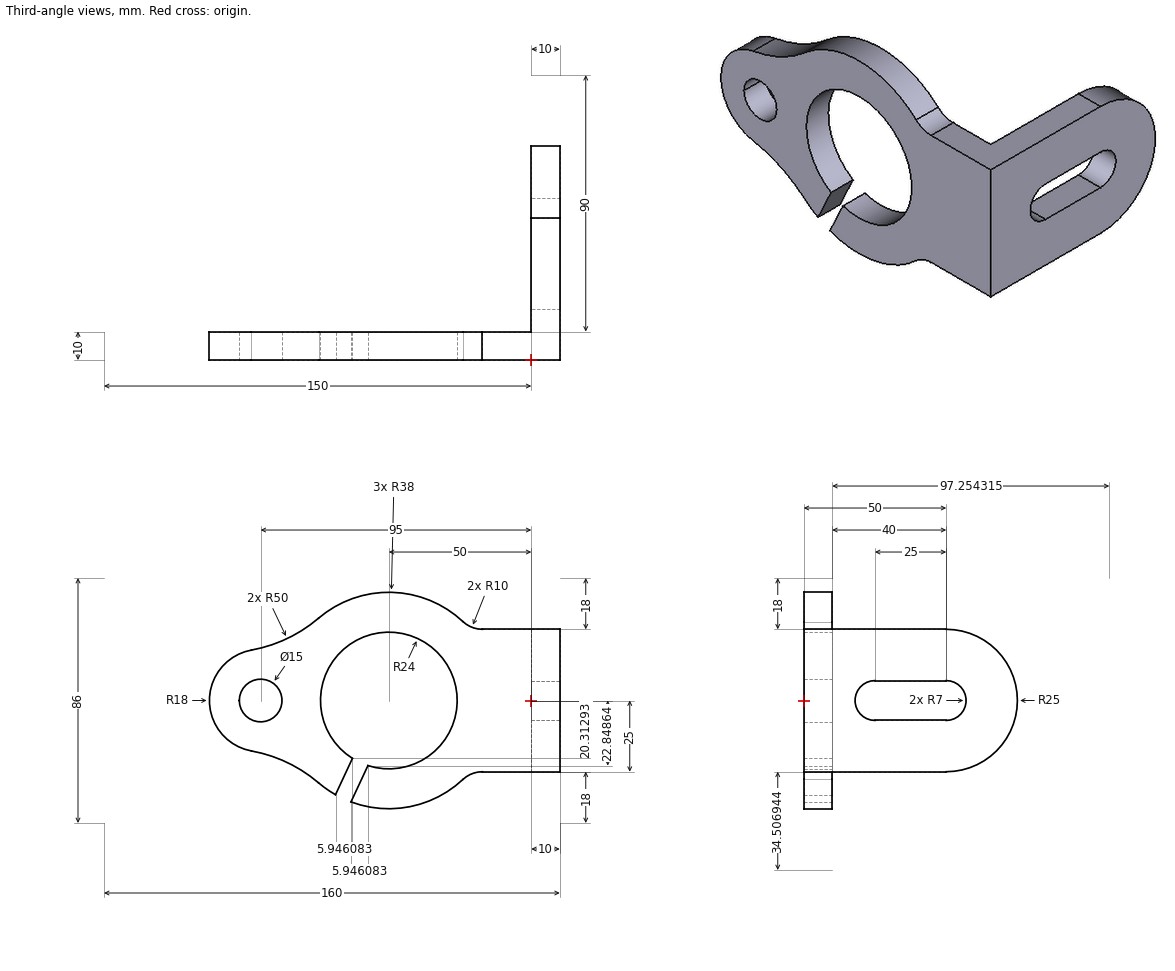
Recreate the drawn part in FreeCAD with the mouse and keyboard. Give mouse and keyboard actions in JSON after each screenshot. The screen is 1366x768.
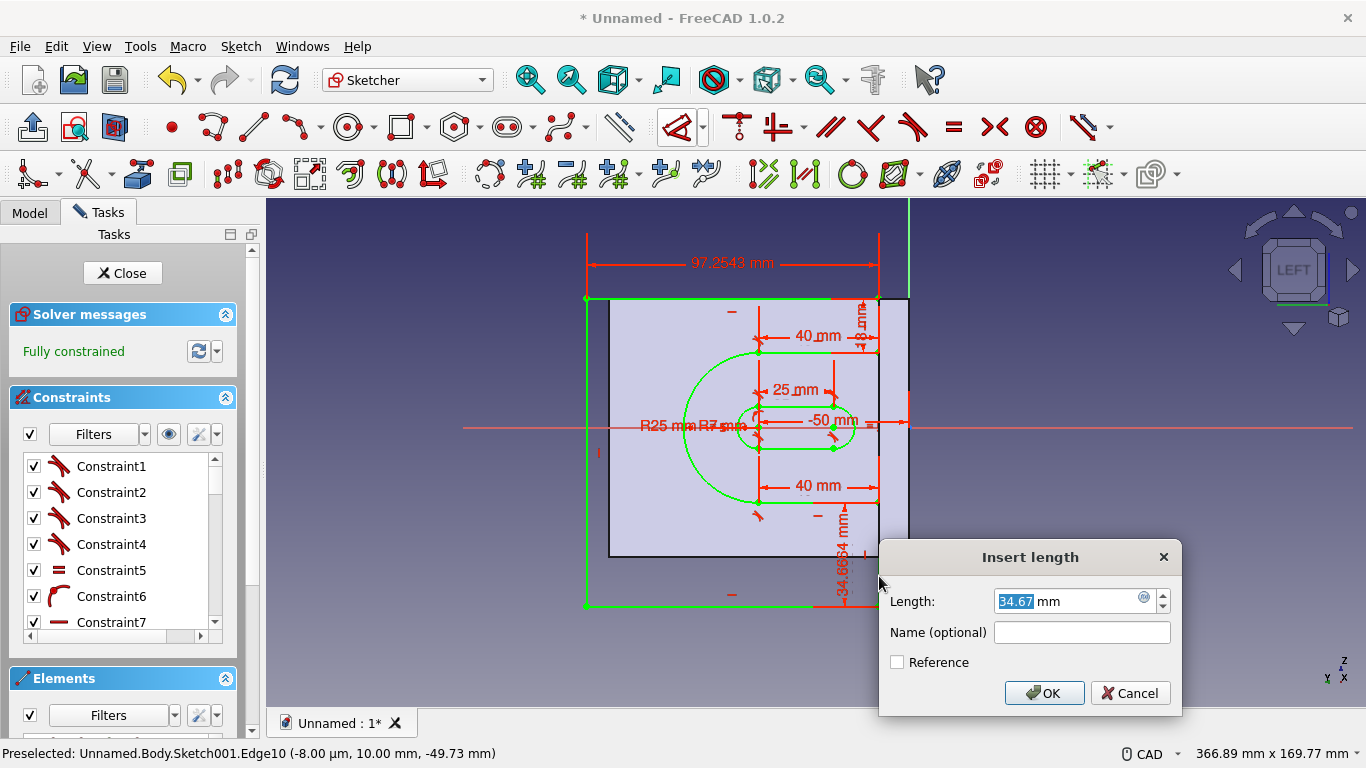
{"action": "type", "text": "34.506944"}
{"action": "key", "text": "Return"}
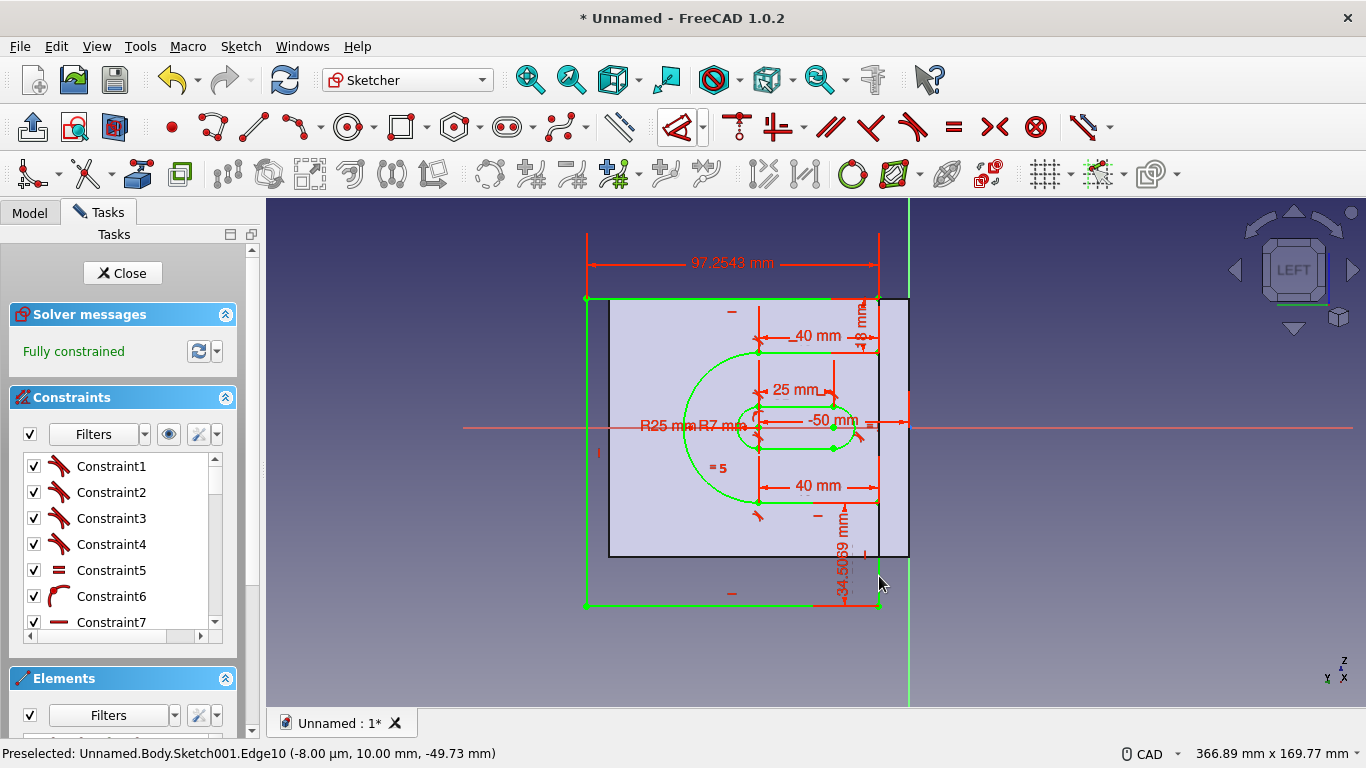
{"action": "left_click", "coordinate": [123, 273]}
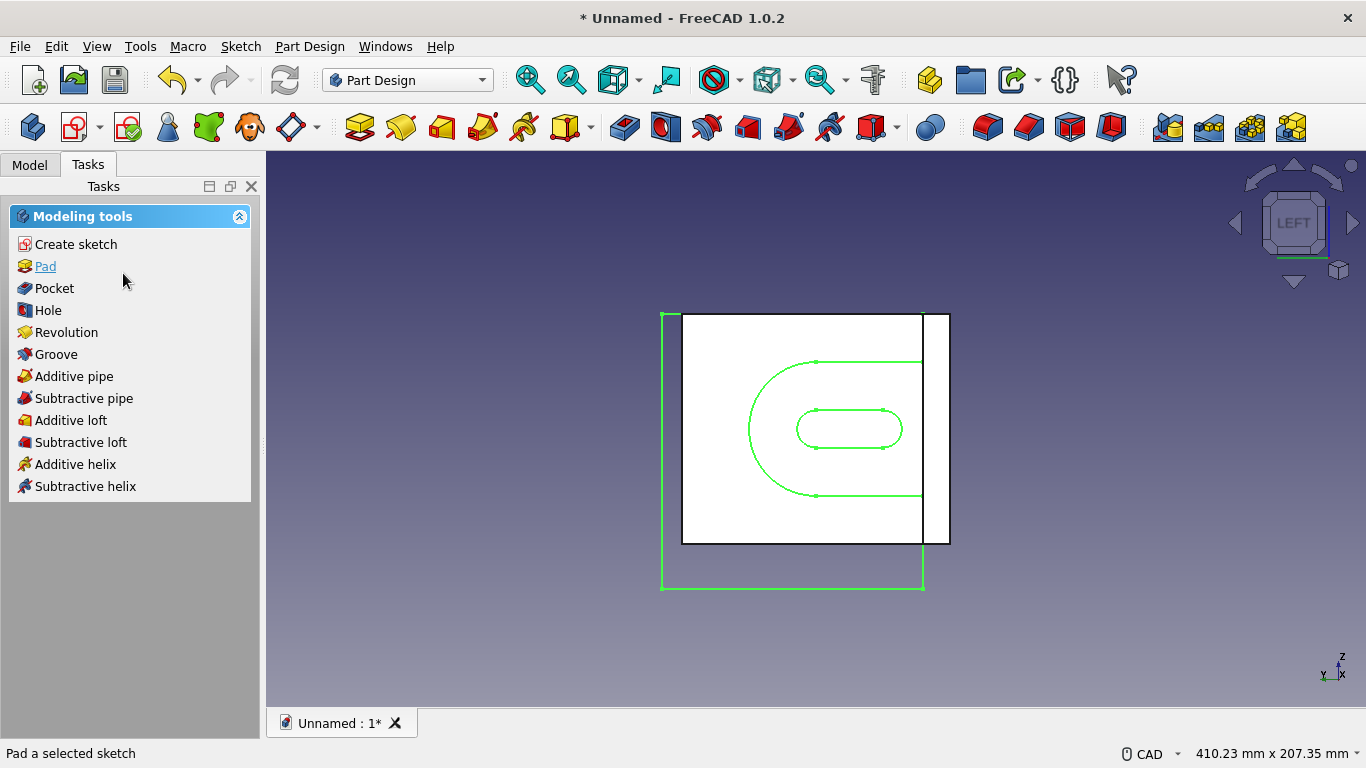
{"action": "left_click", "coordinate": [625, 128]}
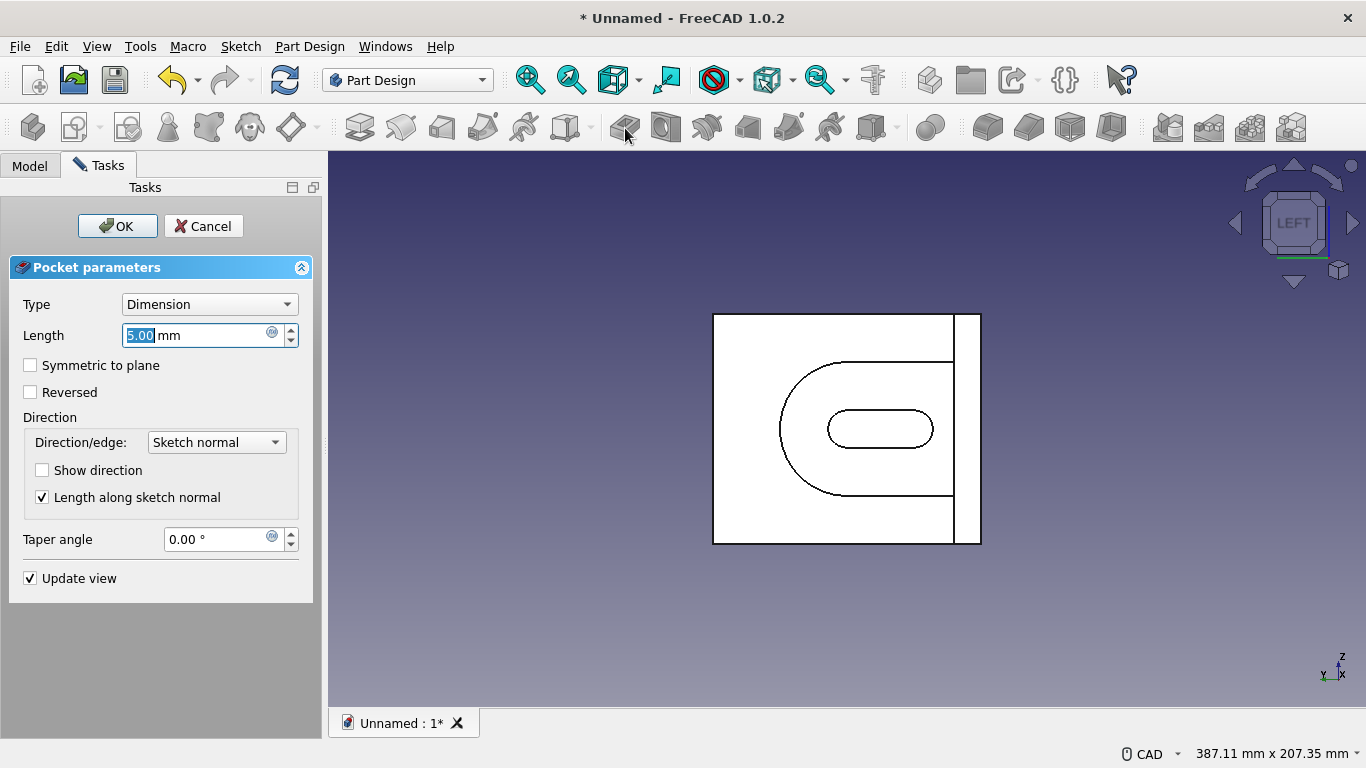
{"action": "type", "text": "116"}
{"action": "key", "text": "Tab"}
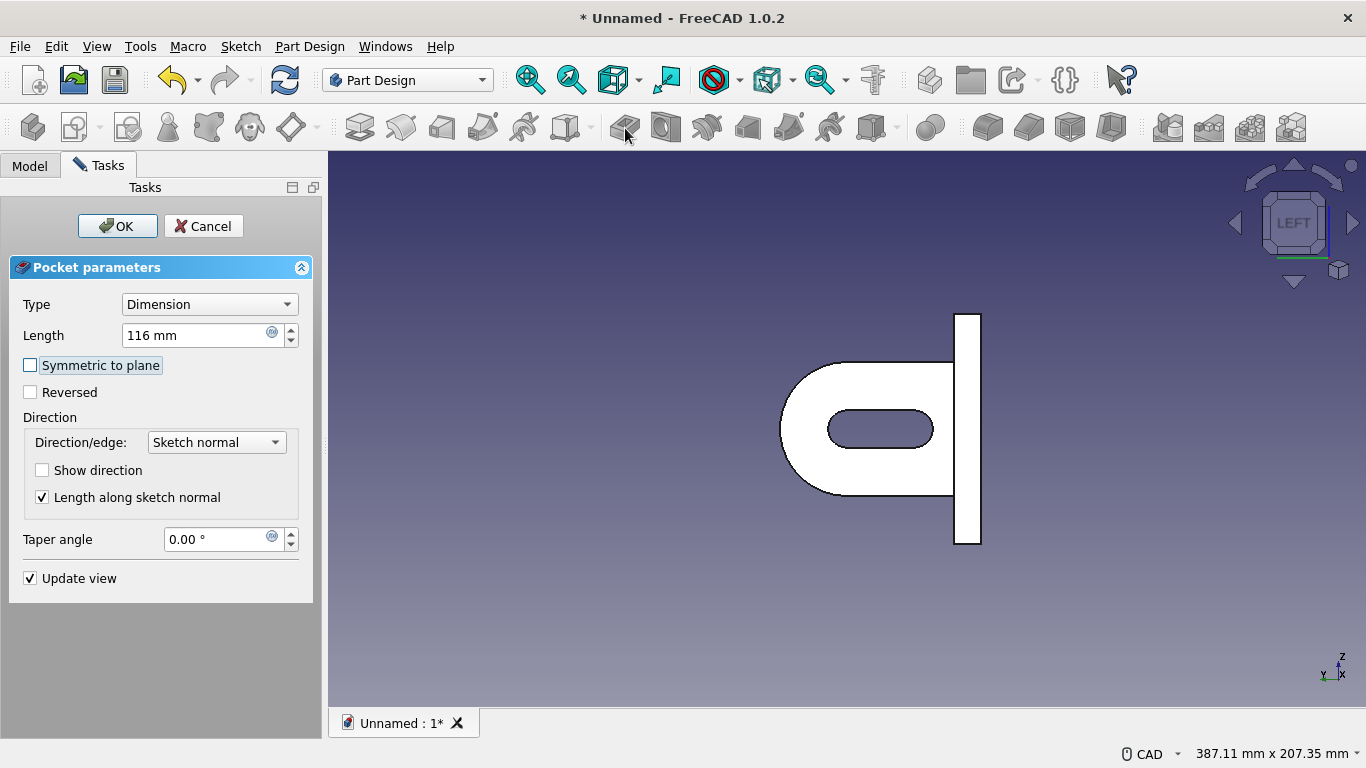
{"action": "left_click", "coordinate": [118, 226]}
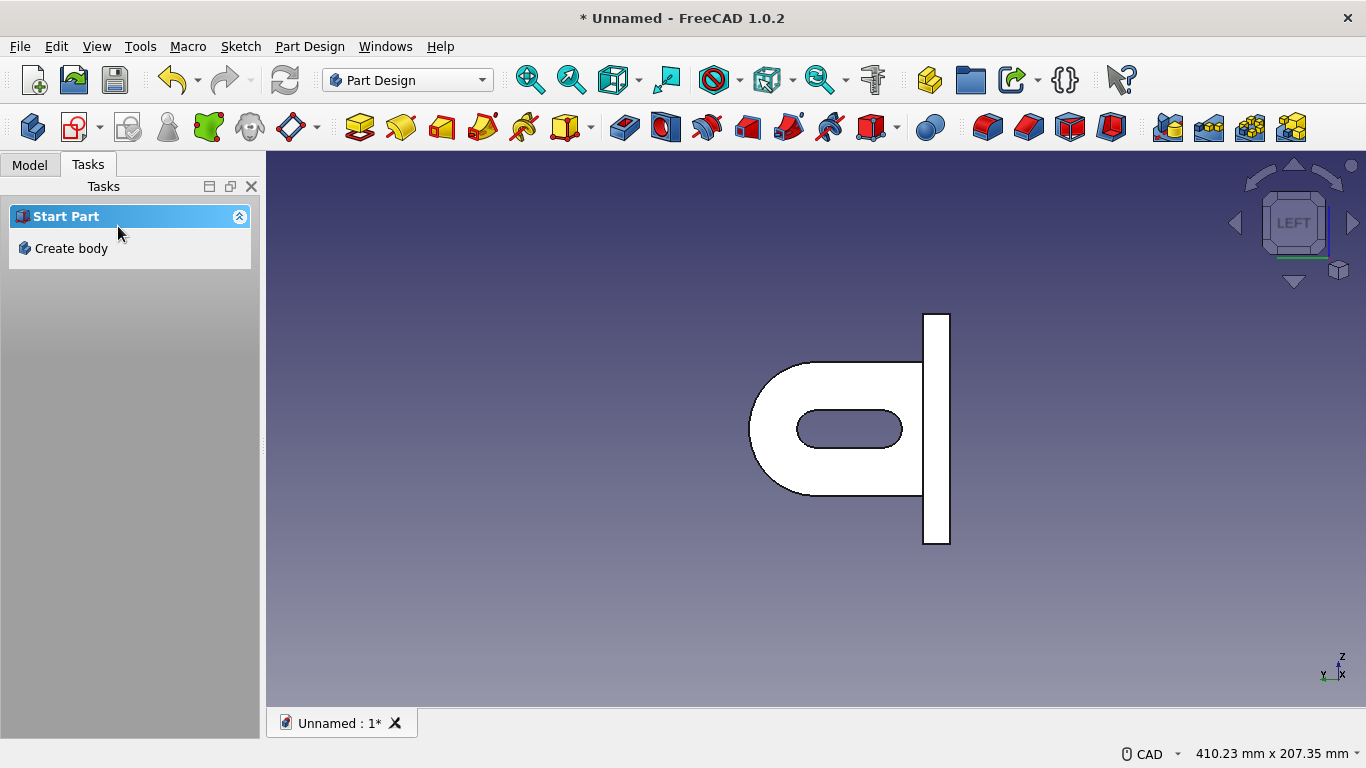
{"action": "key", "text": "v f"}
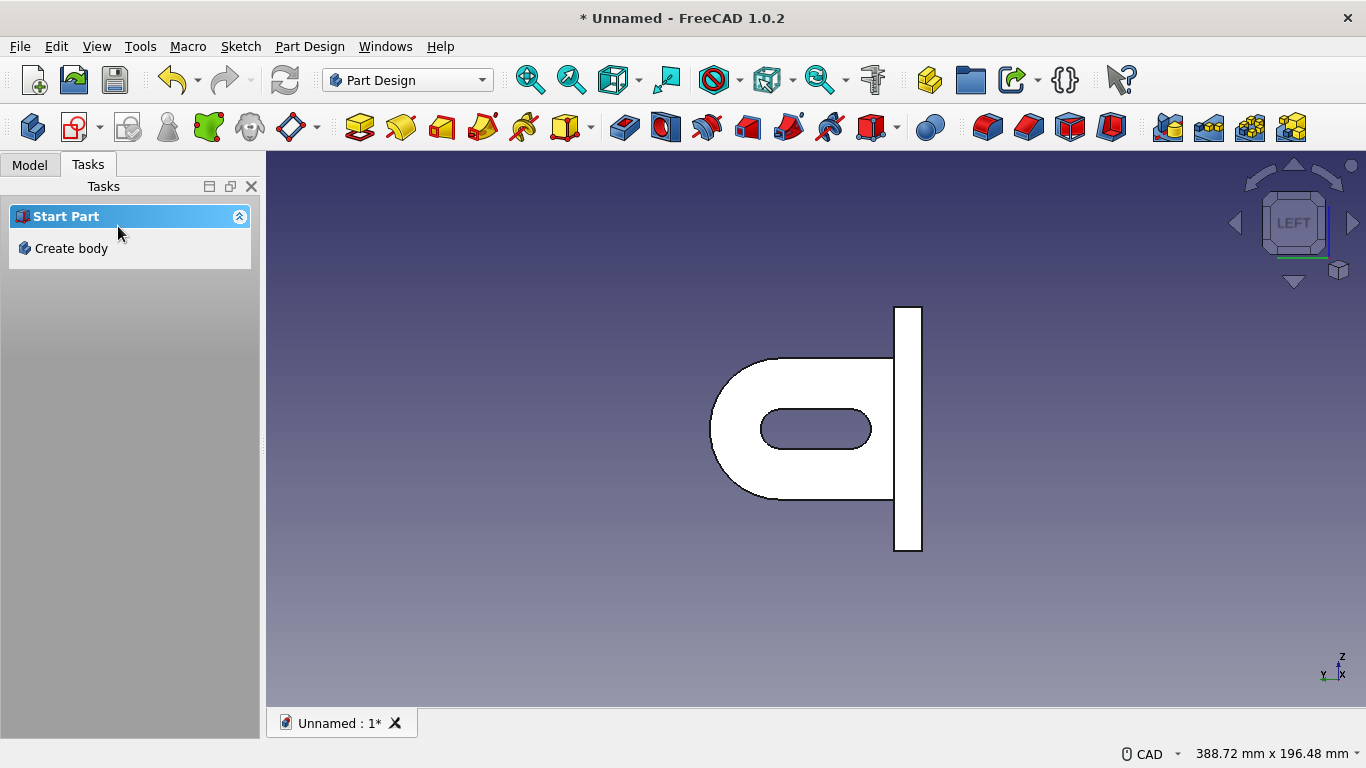
{"action": "key", "text": "4"}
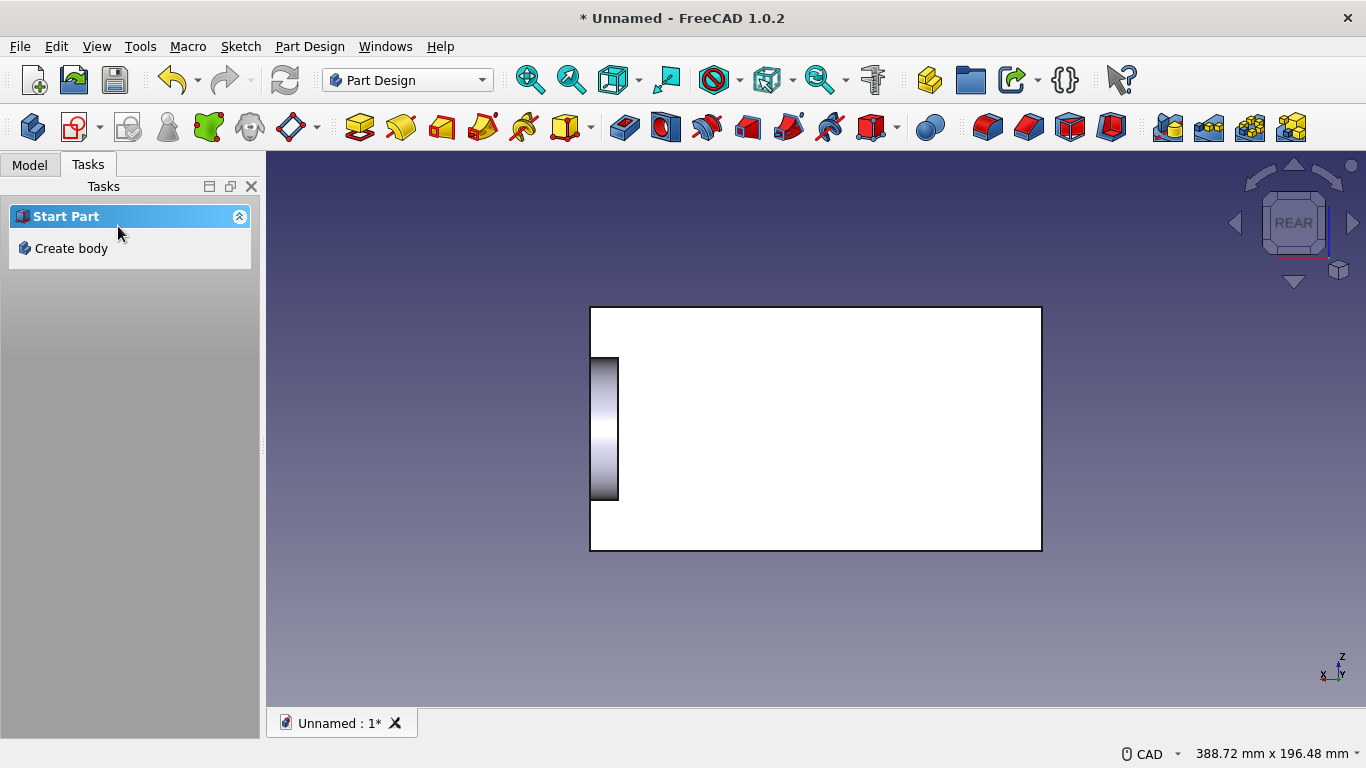
{"action": "key", "text": "v f"}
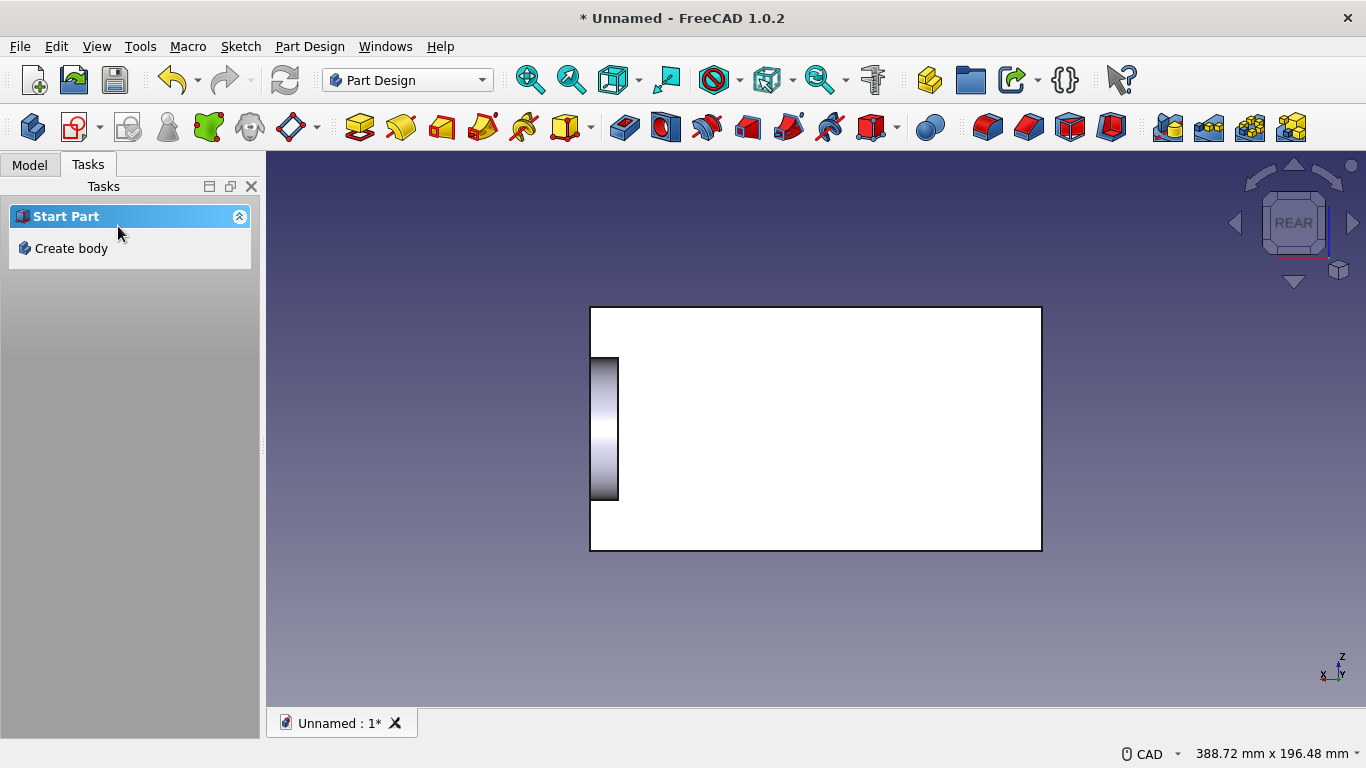
{"action": "left_click", "coordinate": [751, 428]}